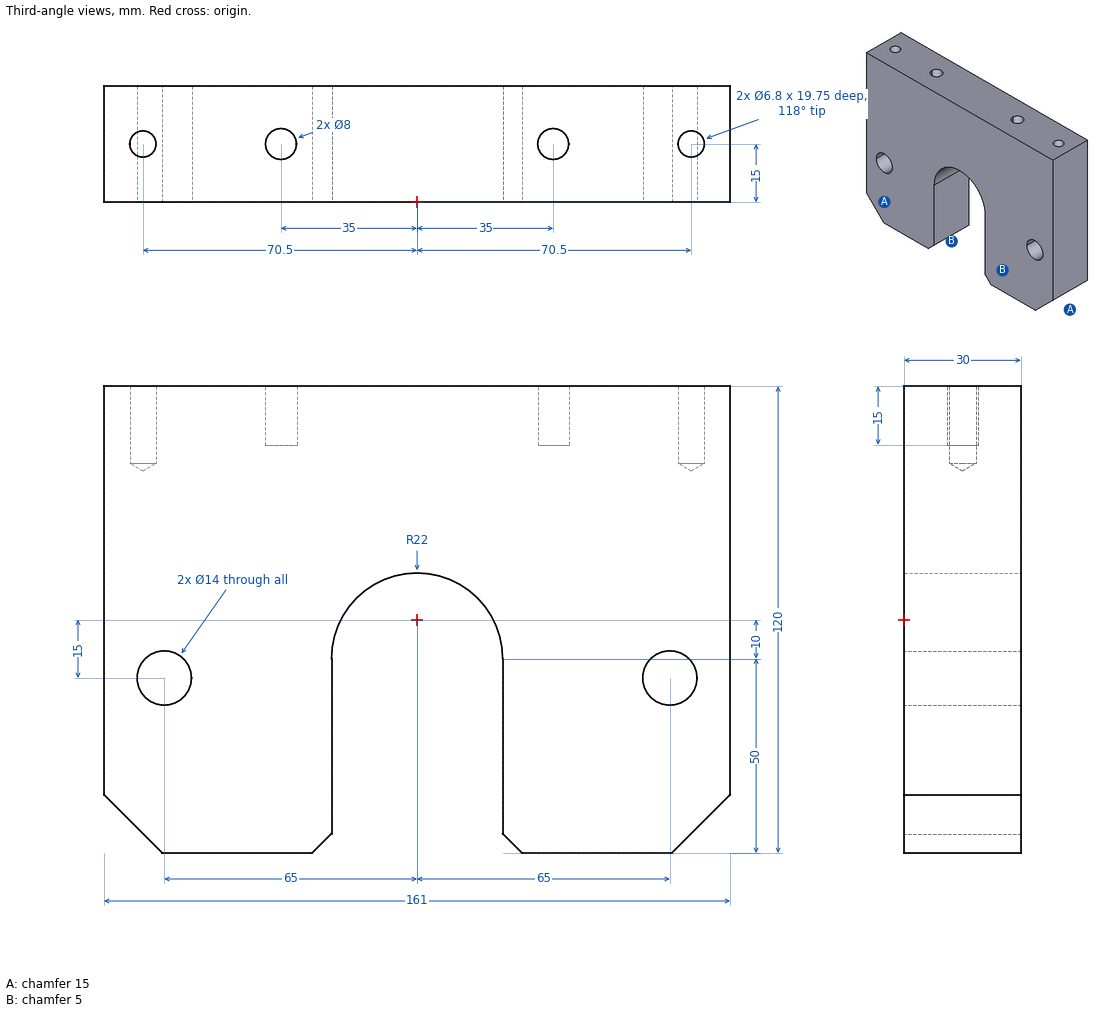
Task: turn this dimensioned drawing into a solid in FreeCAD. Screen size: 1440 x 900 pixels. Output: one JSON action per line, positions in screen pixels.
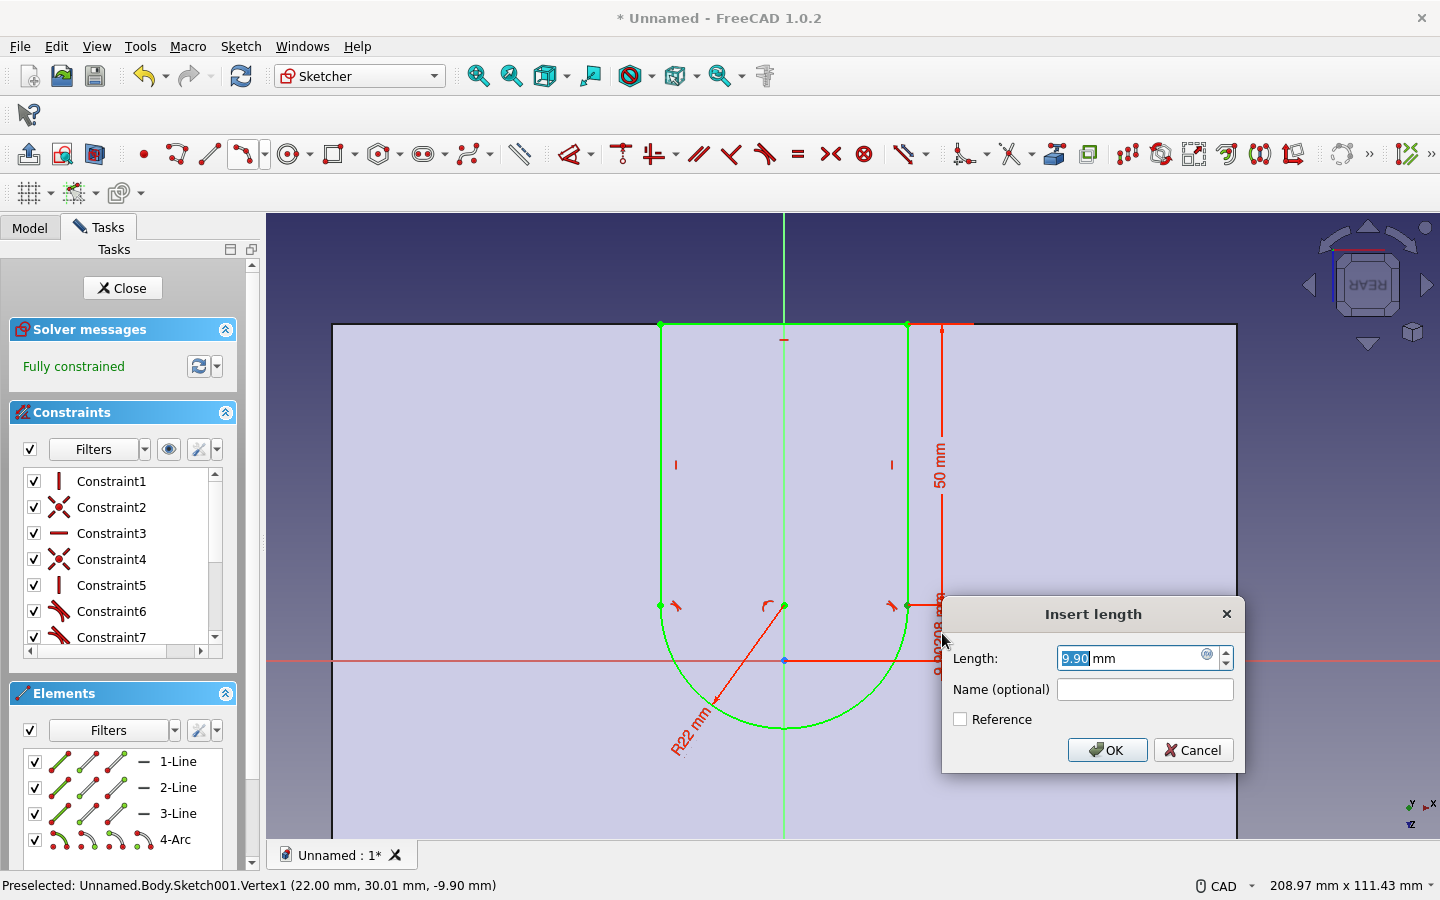
{"action": "type", "text": "10"}
{"action": "key", "text": "Return"}
{"action": "key", "text": "Escape"}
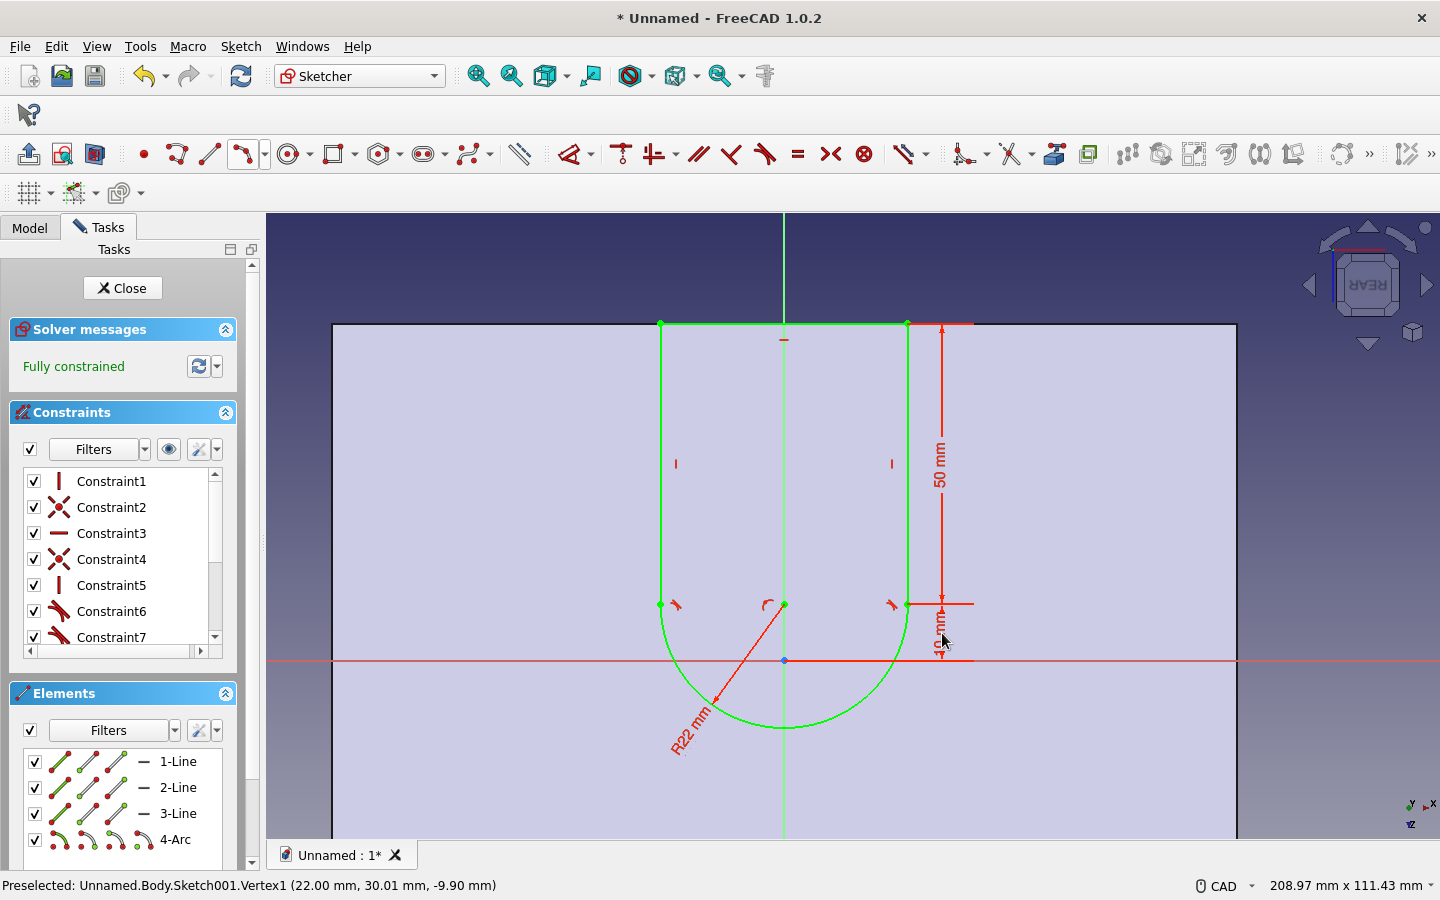
{"action": "left_click", "coordinate": [123, 288]}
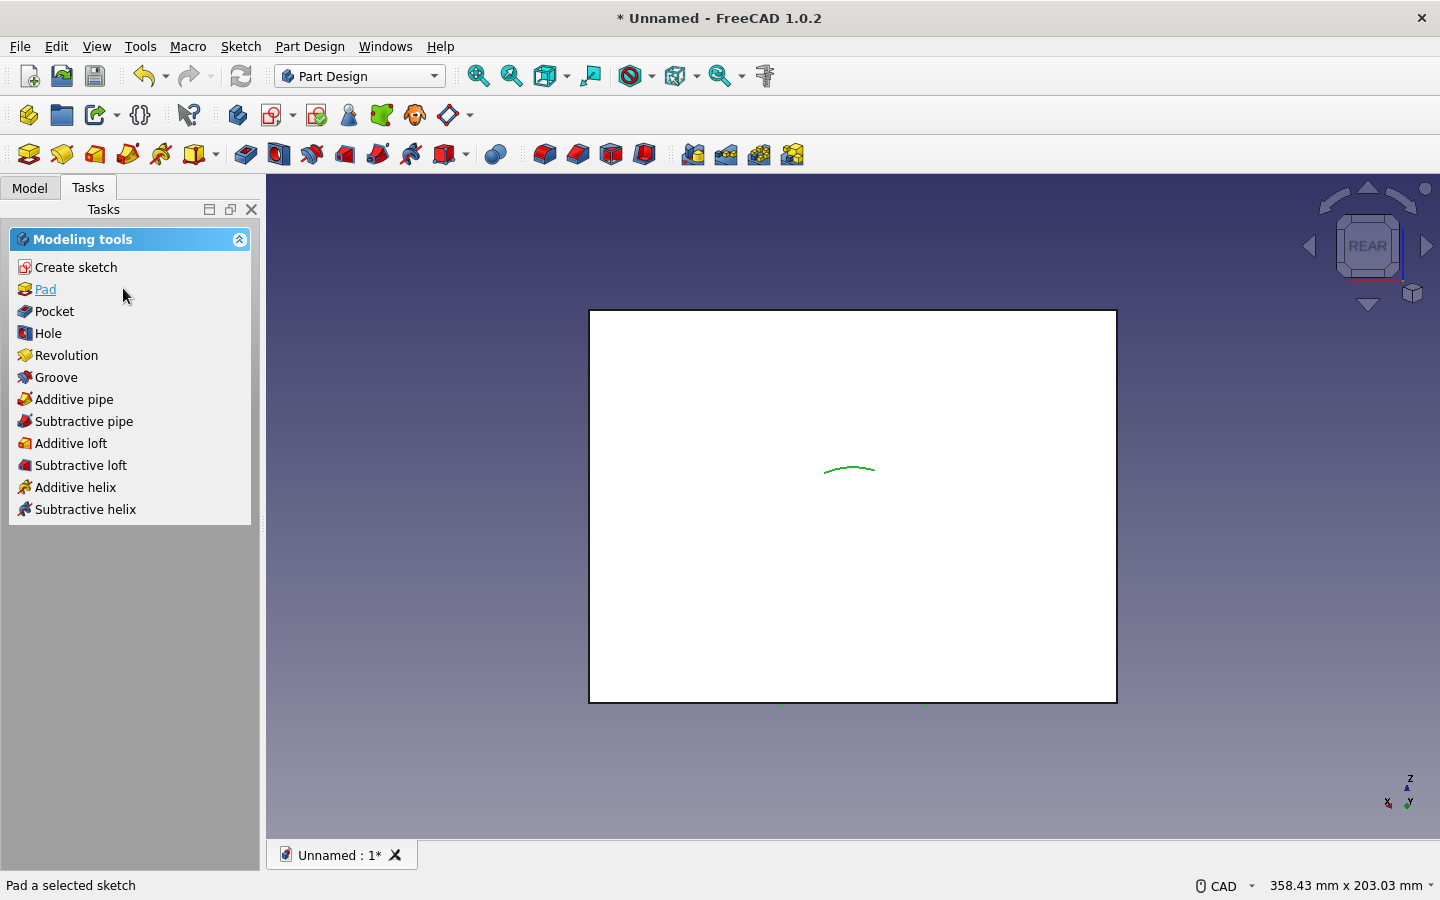
{"action": "left_click", "coordinate": [246, 154]}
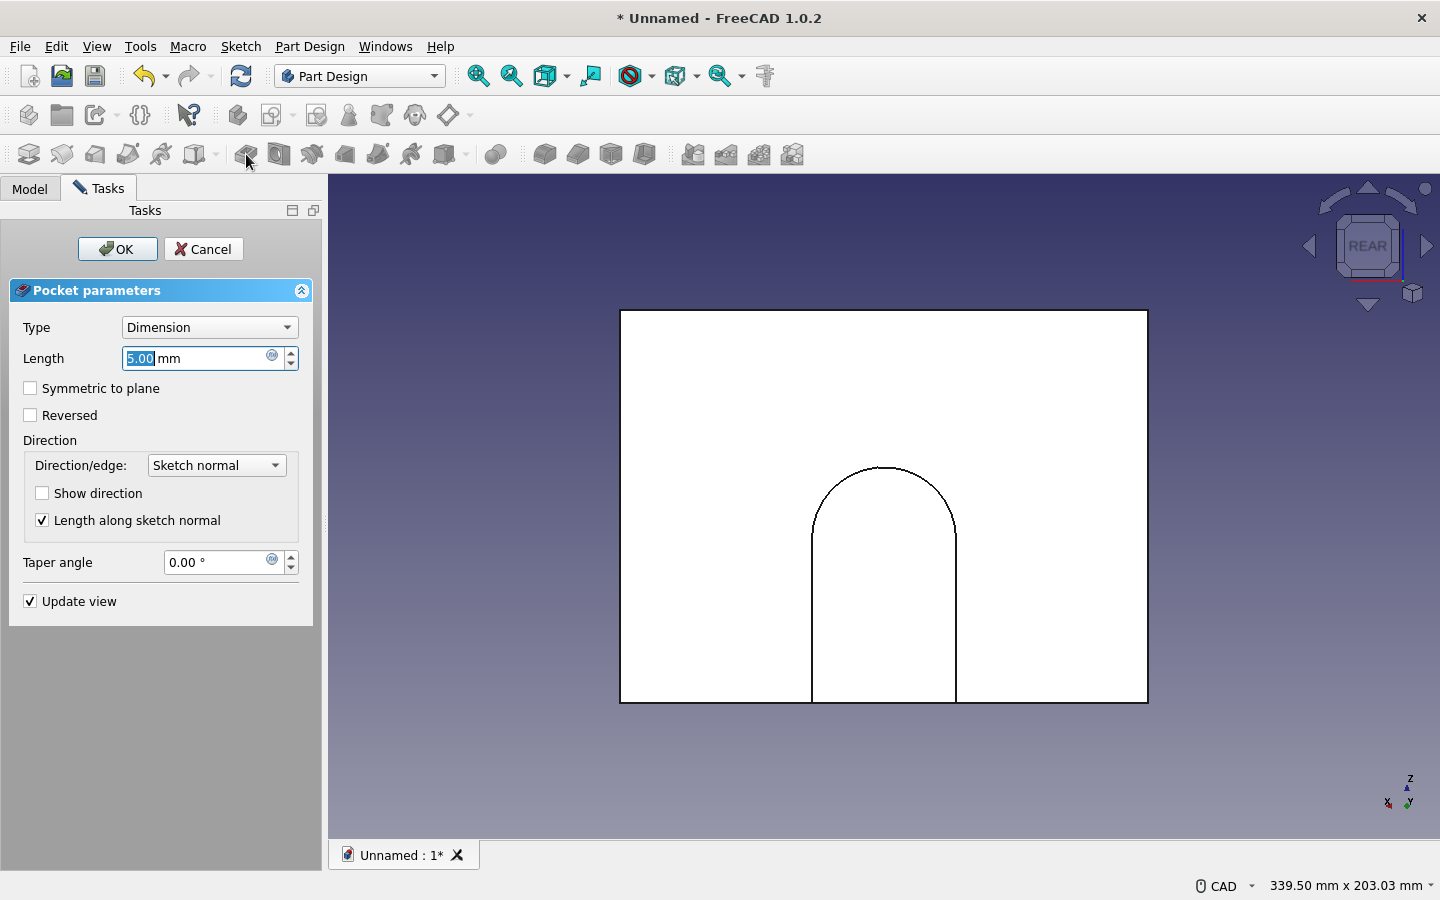
{"action": "left_click", "coordinate": [210, 328]}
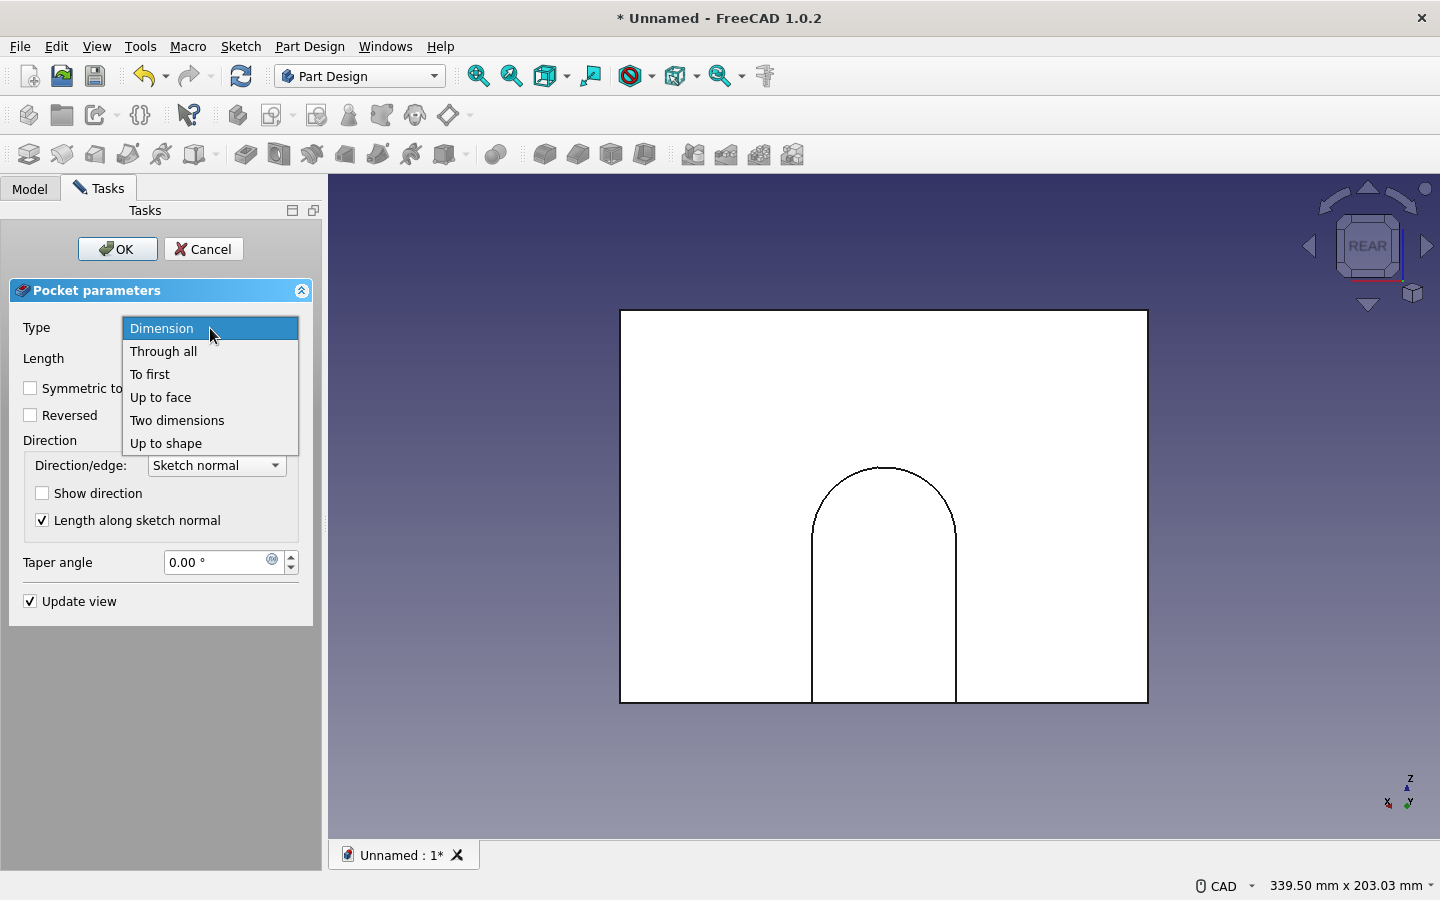
{"action": "left_click", "coordinate": [208, 352]}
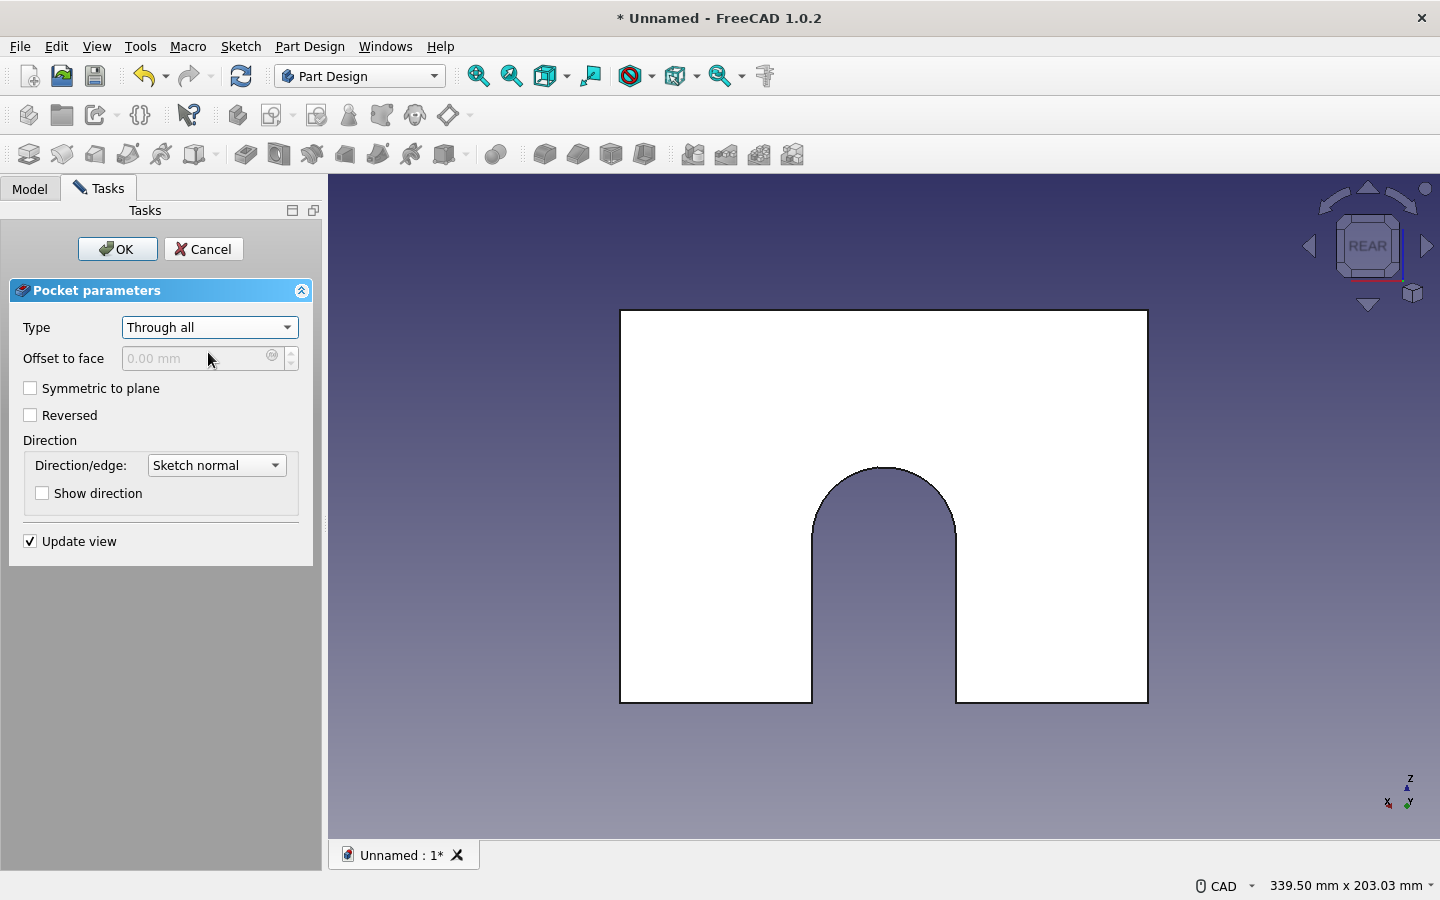
{"action": "left_click", "coordinate": [118, 249]}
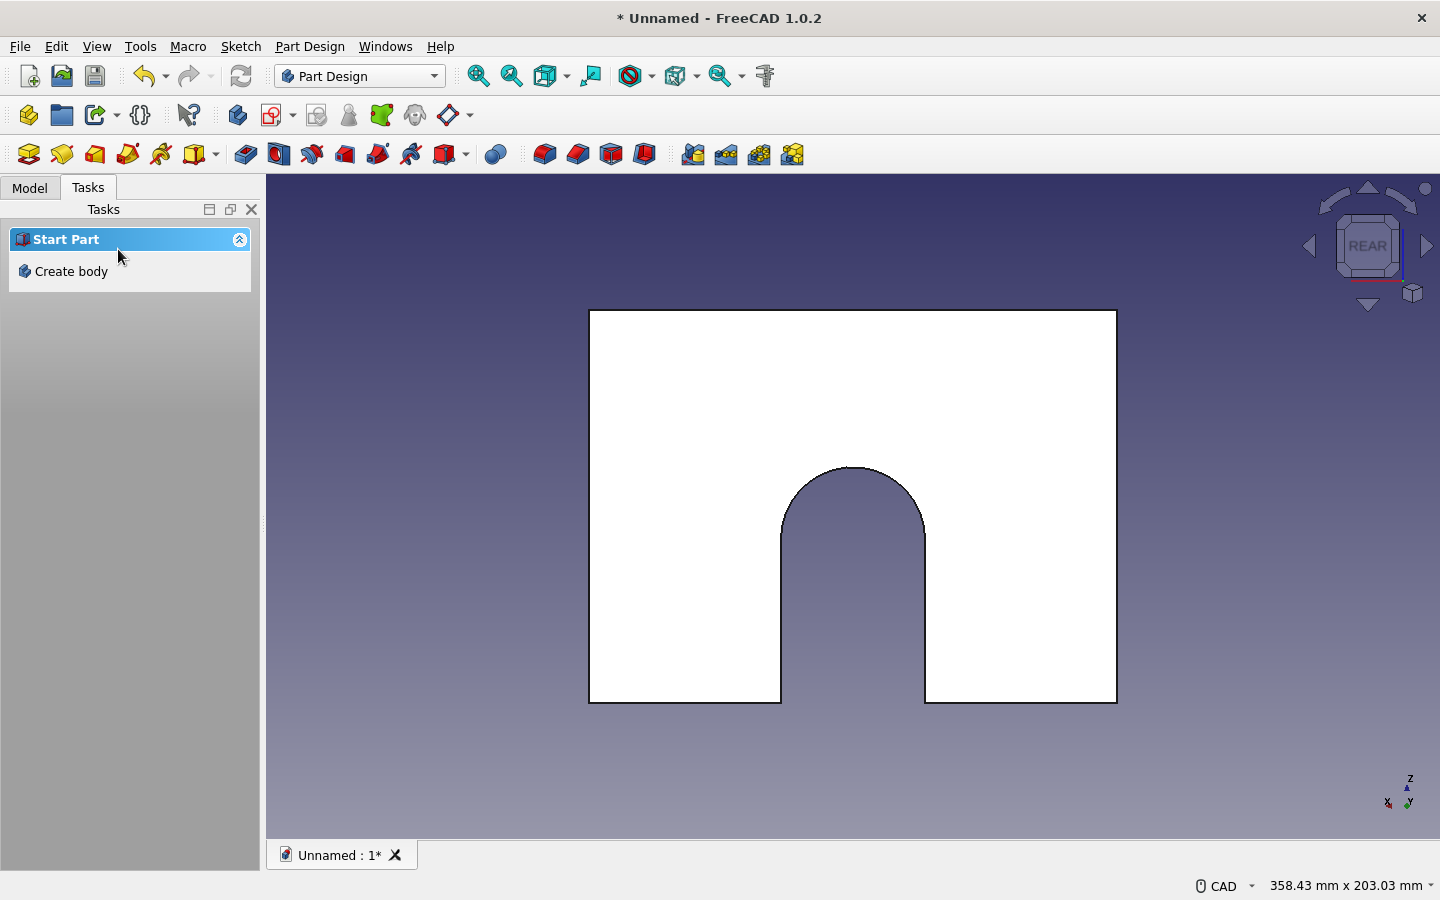
{"action": "left_click", "coordinate": [702, 449]}